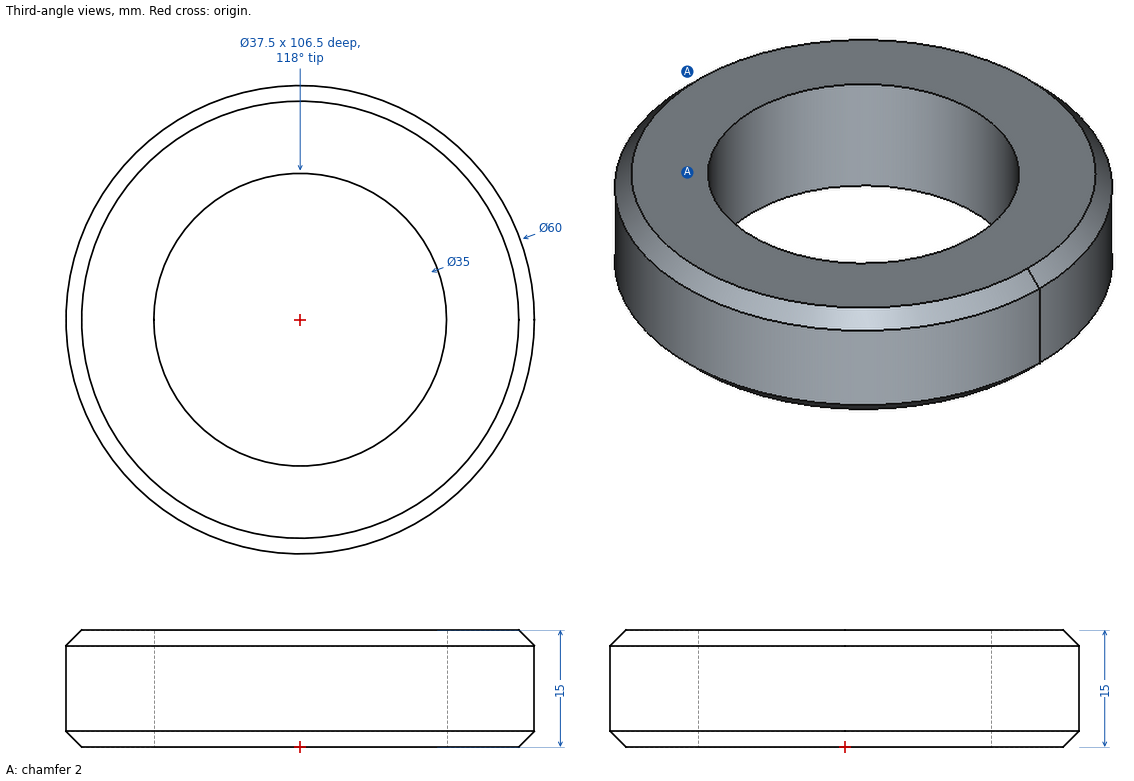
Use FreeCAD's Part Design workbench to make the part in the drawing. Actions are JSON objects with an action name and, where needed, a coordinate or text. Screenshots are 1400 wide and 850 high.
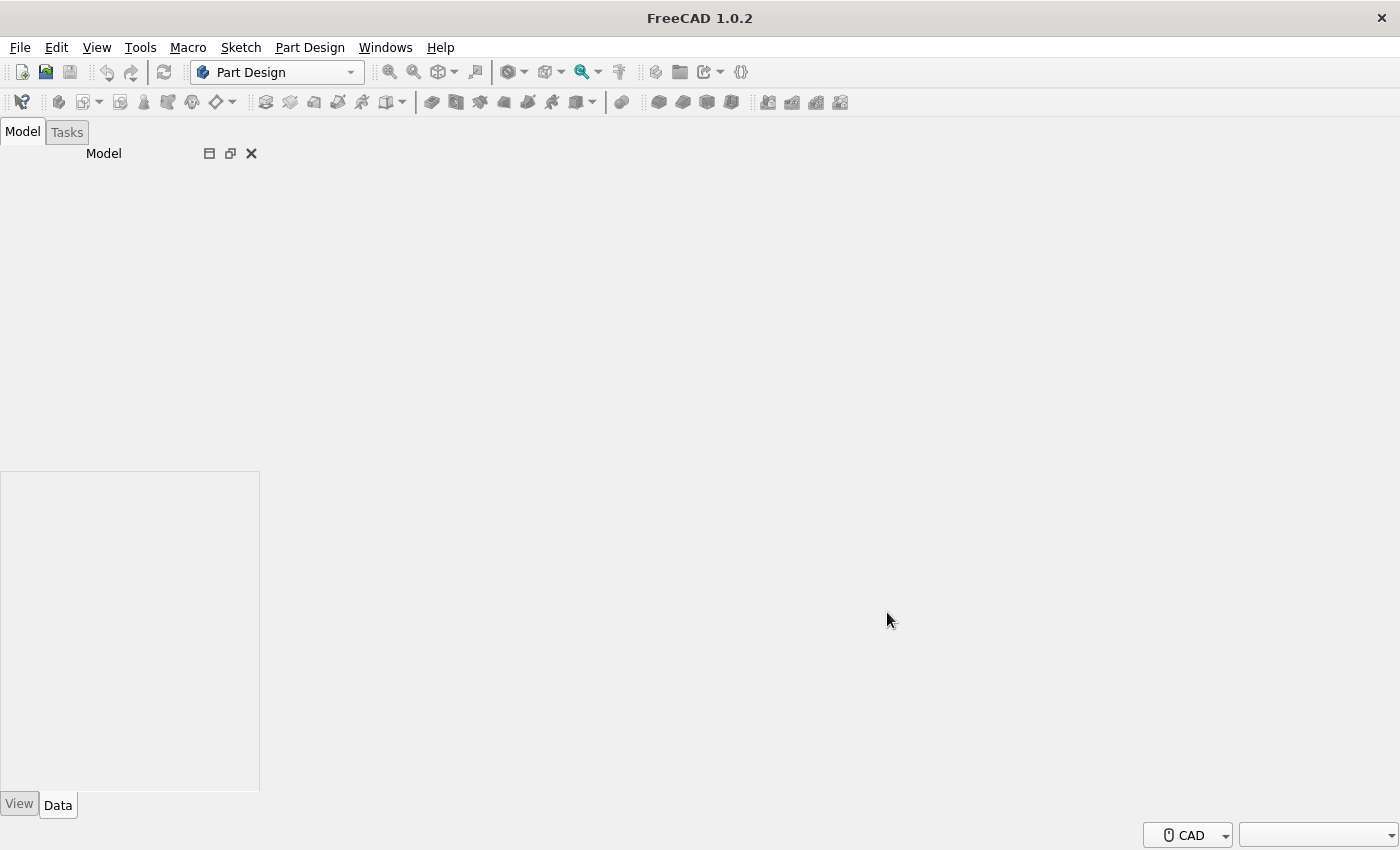
{"action": "left_click", "coordinate": [22, 72]}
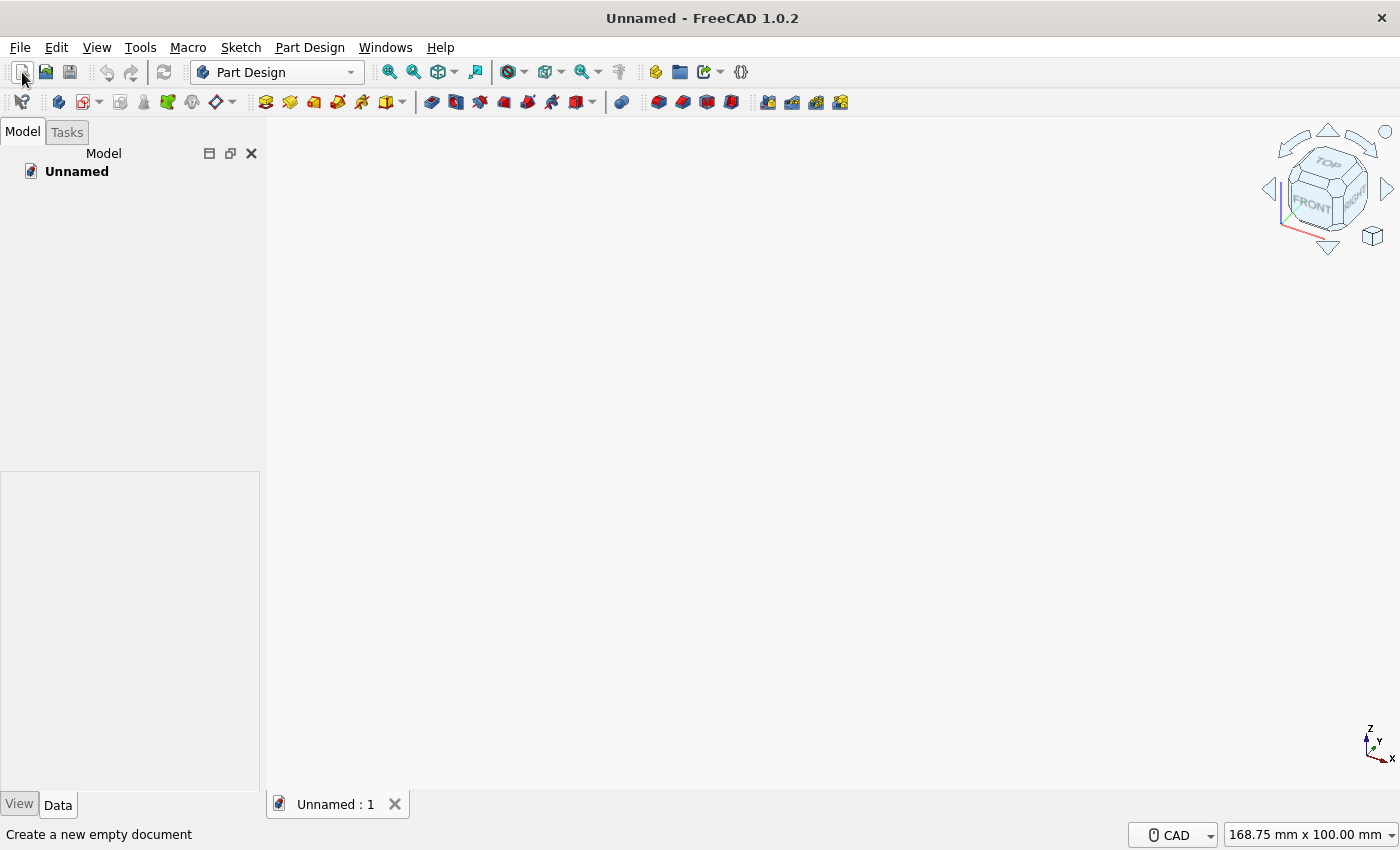
{"action": "left_click", "coordinate": [84, 102]}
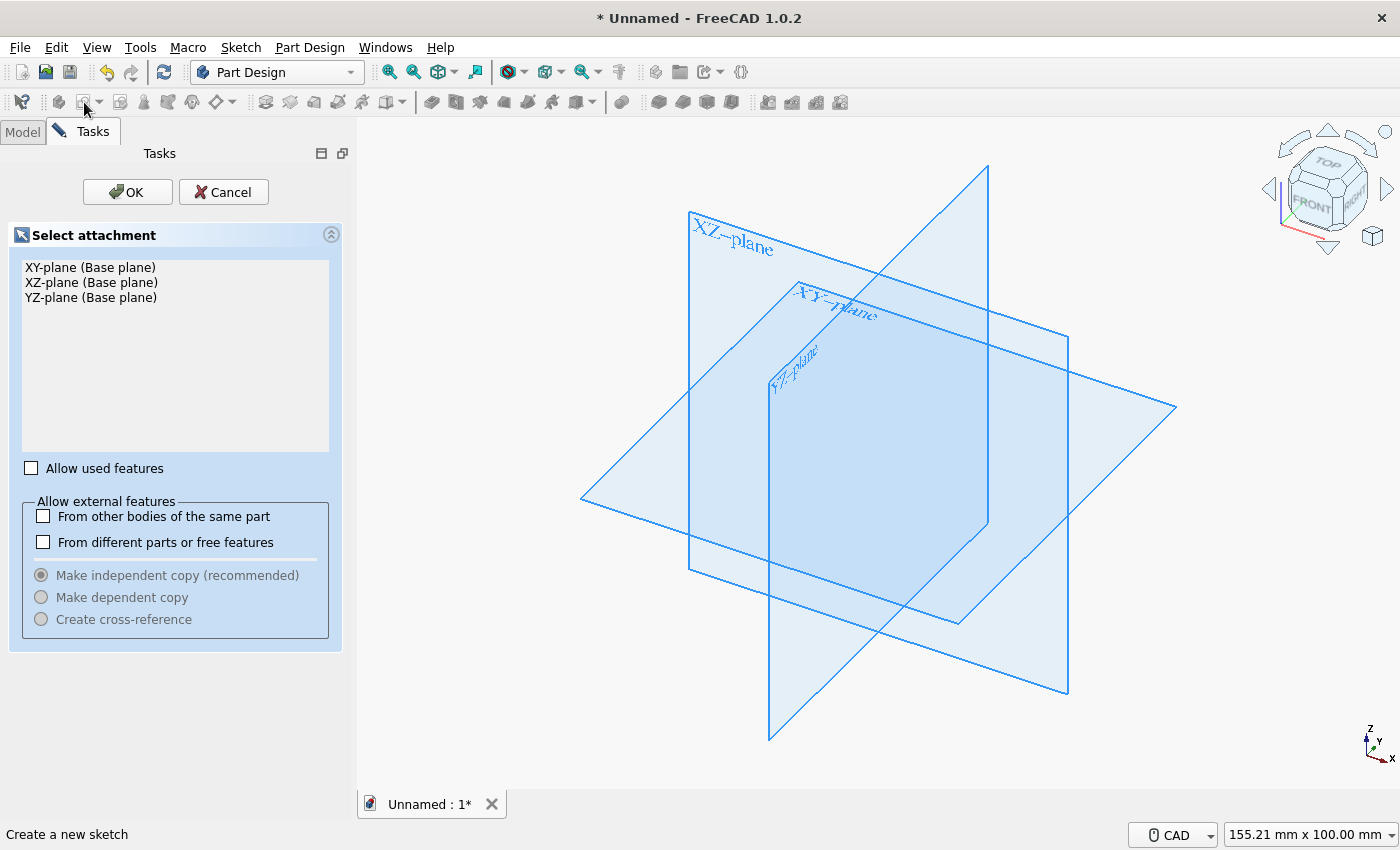
{"action": "left_click", "coordinate": [82, 268]}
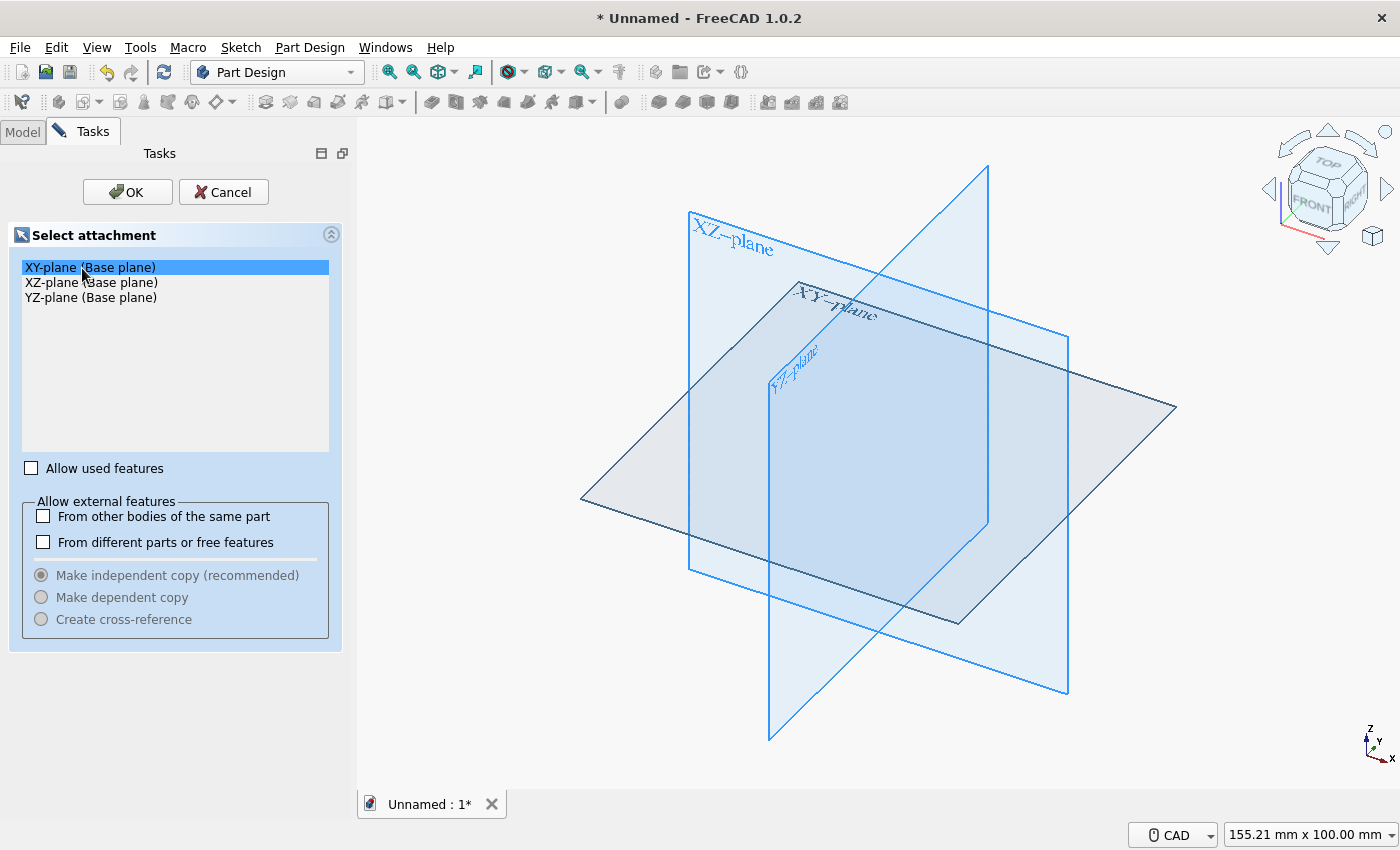
{"action": "left_click", "coordinate": [128, 192]}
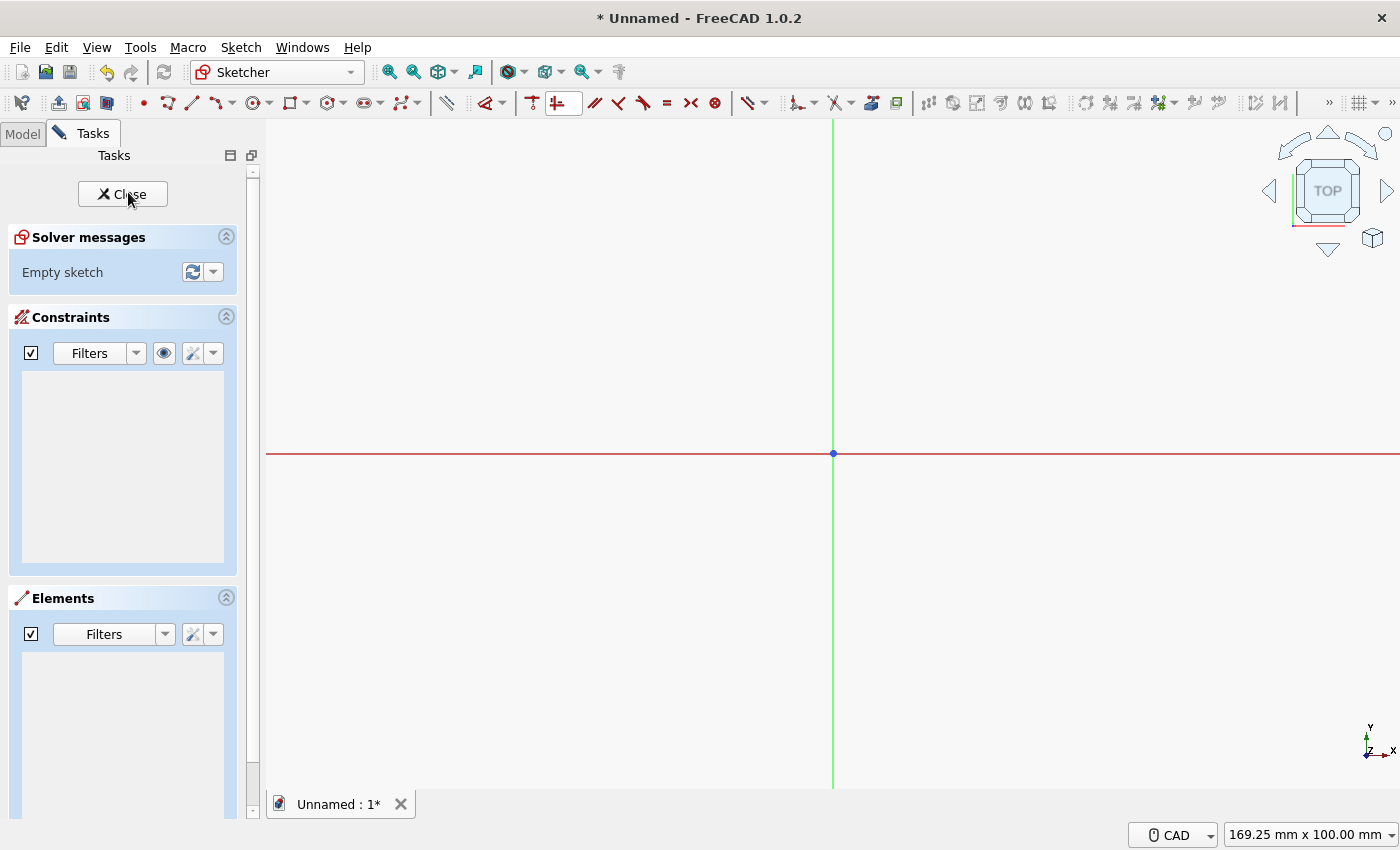
{"action": "left_click", "coordinate": [254, 104]}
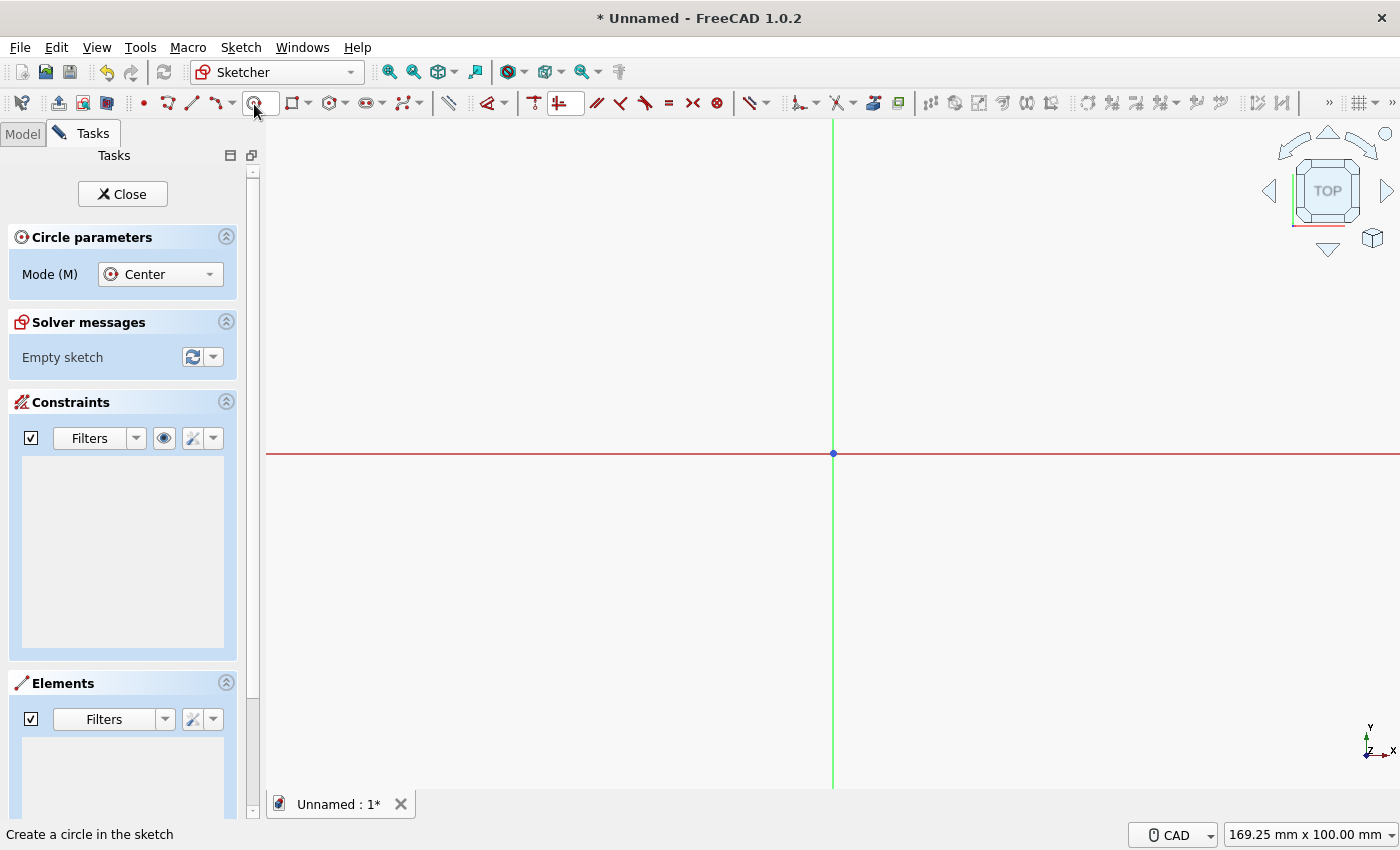
{"action": "left_click", "coordinate": [833, 454]}
{"action": "mouse_move", "coordinate": [975, 312]}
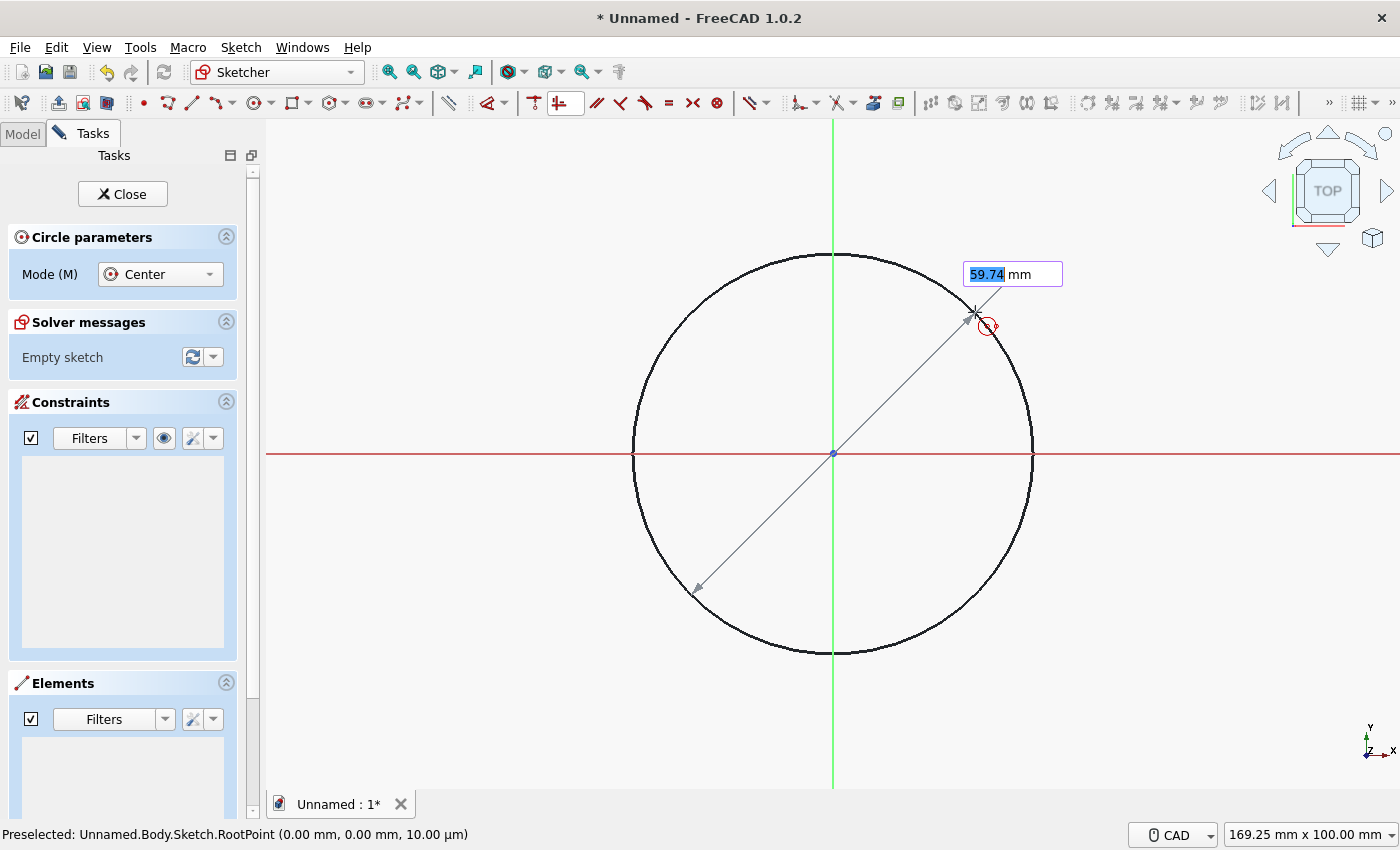
{"action": "type", "text": "60"}
{"action": "key", "text": "Return"}
{"action": "key", "text": "Escape"}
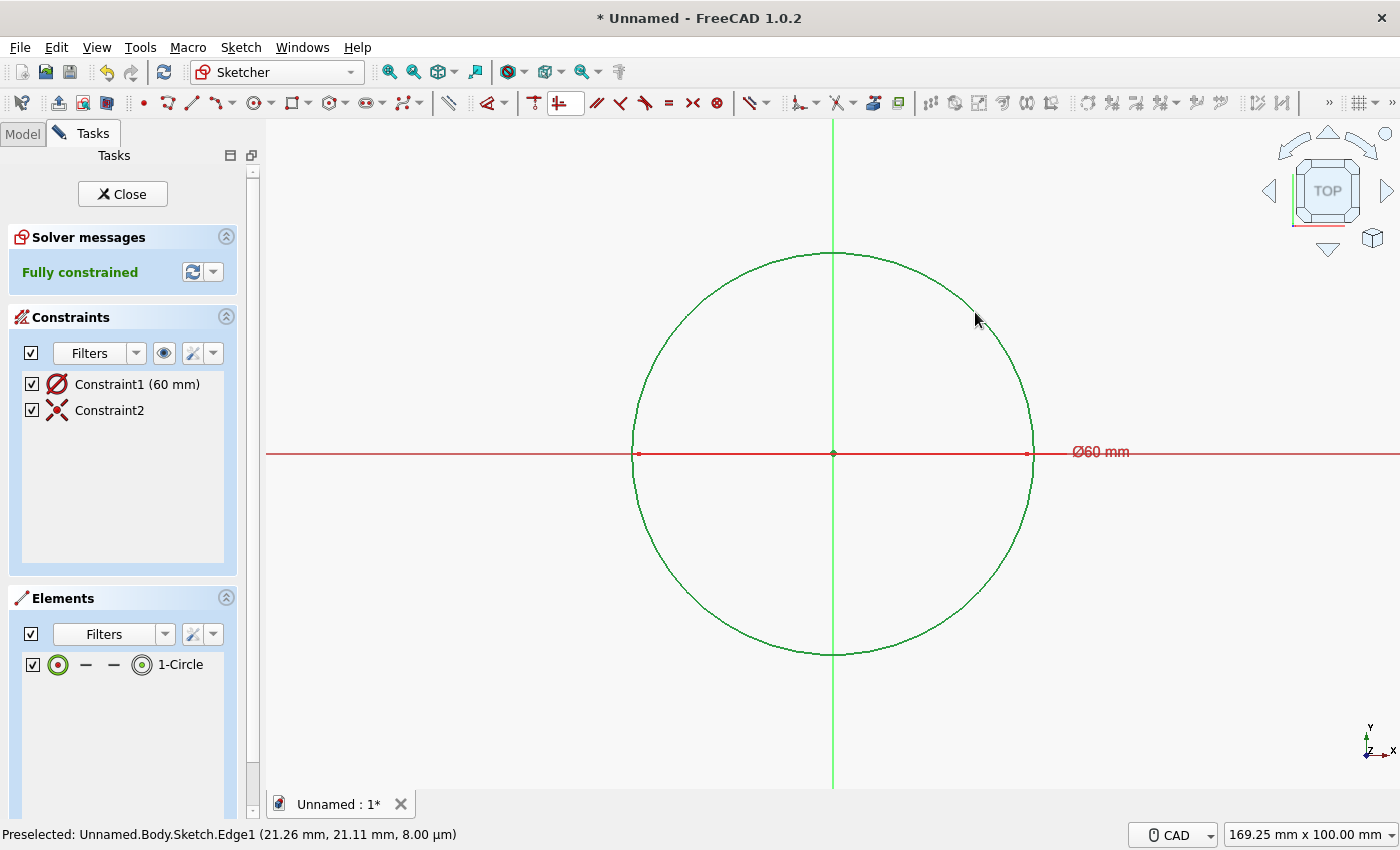
{"action": "left_click", "coordinate": [123, 194]}